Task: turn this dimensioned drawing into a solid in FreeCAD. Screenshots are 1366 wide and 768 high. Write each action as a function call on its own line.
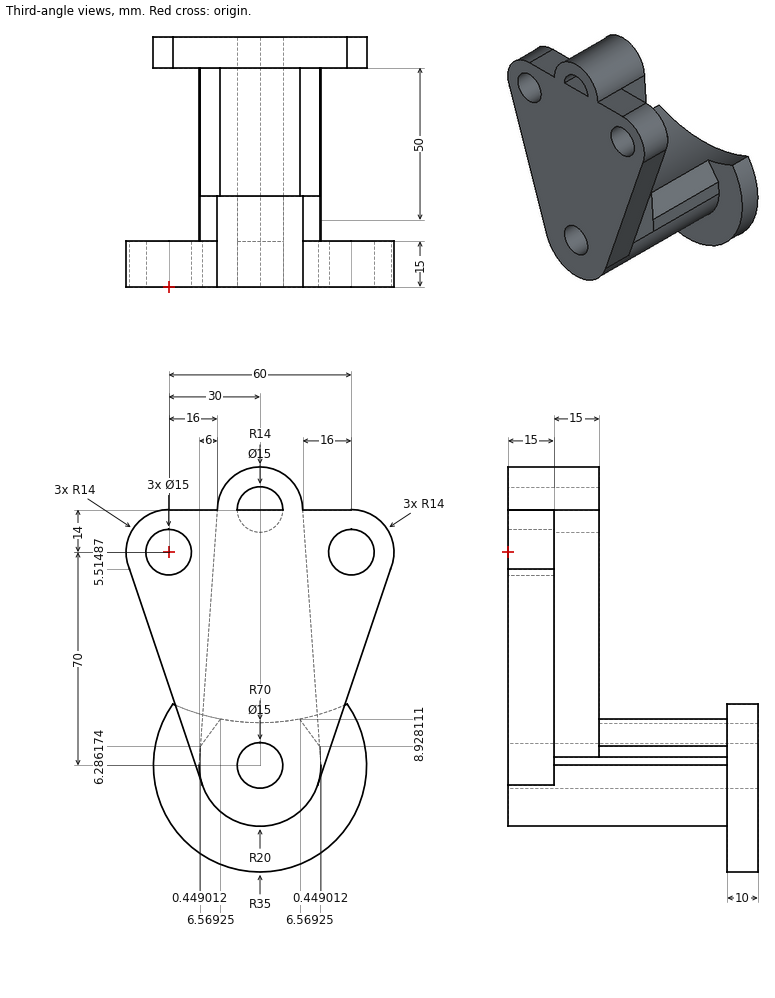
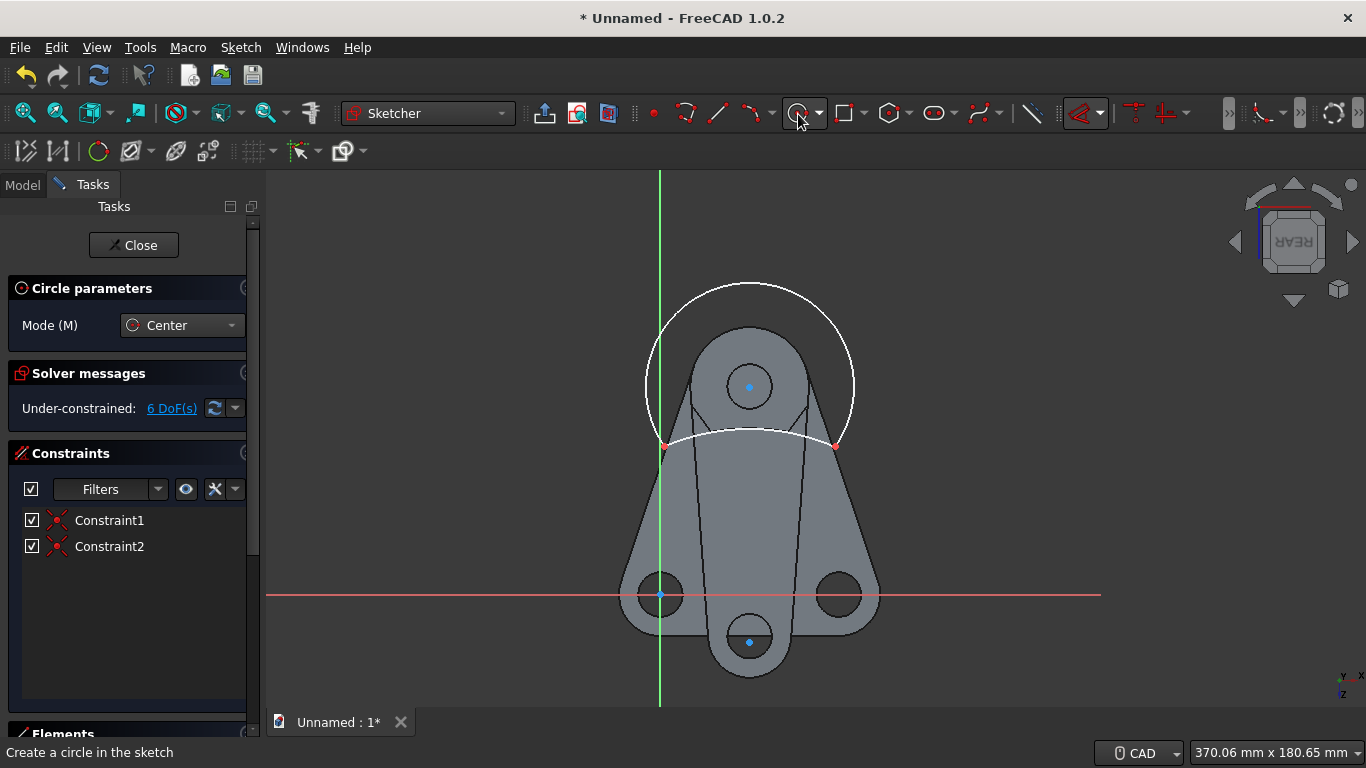
click(750, 387)
move(765, 371)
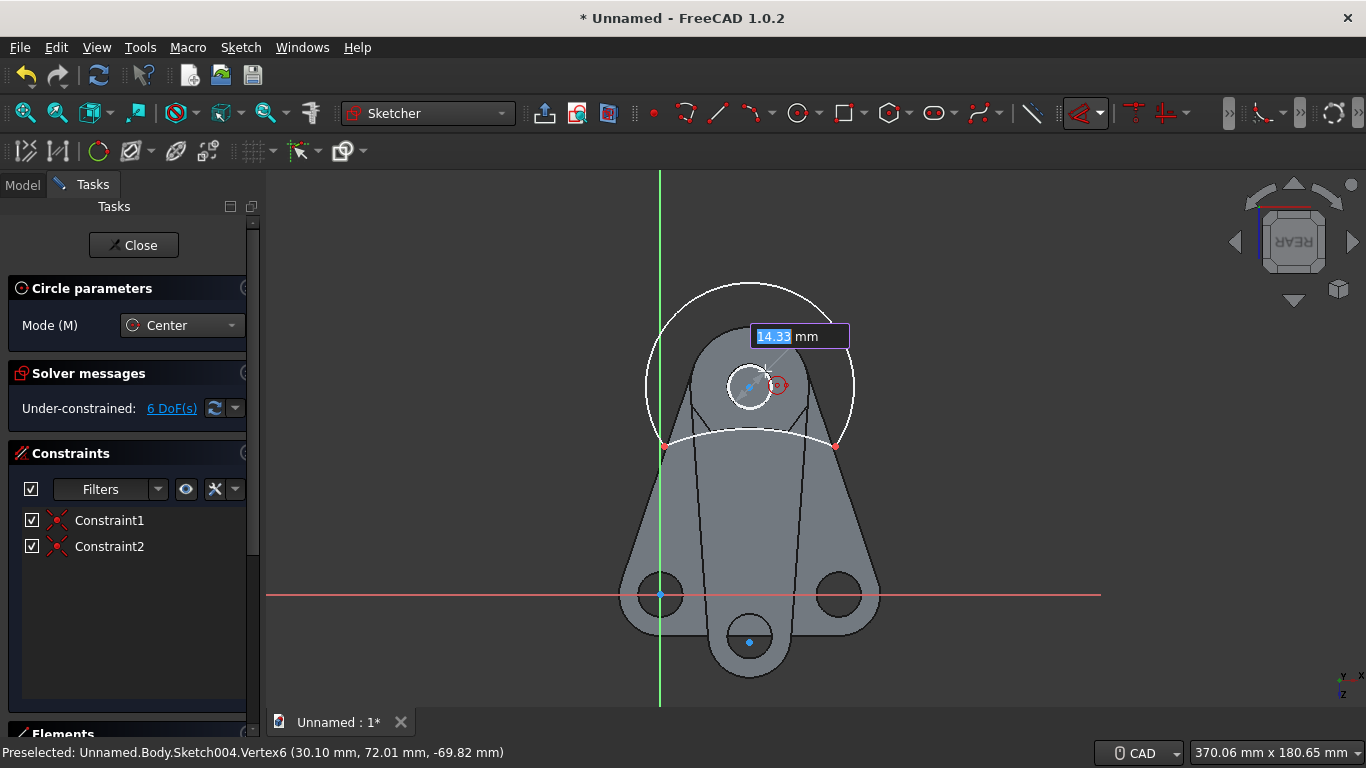
text(15)
key(Return)
key(Escape)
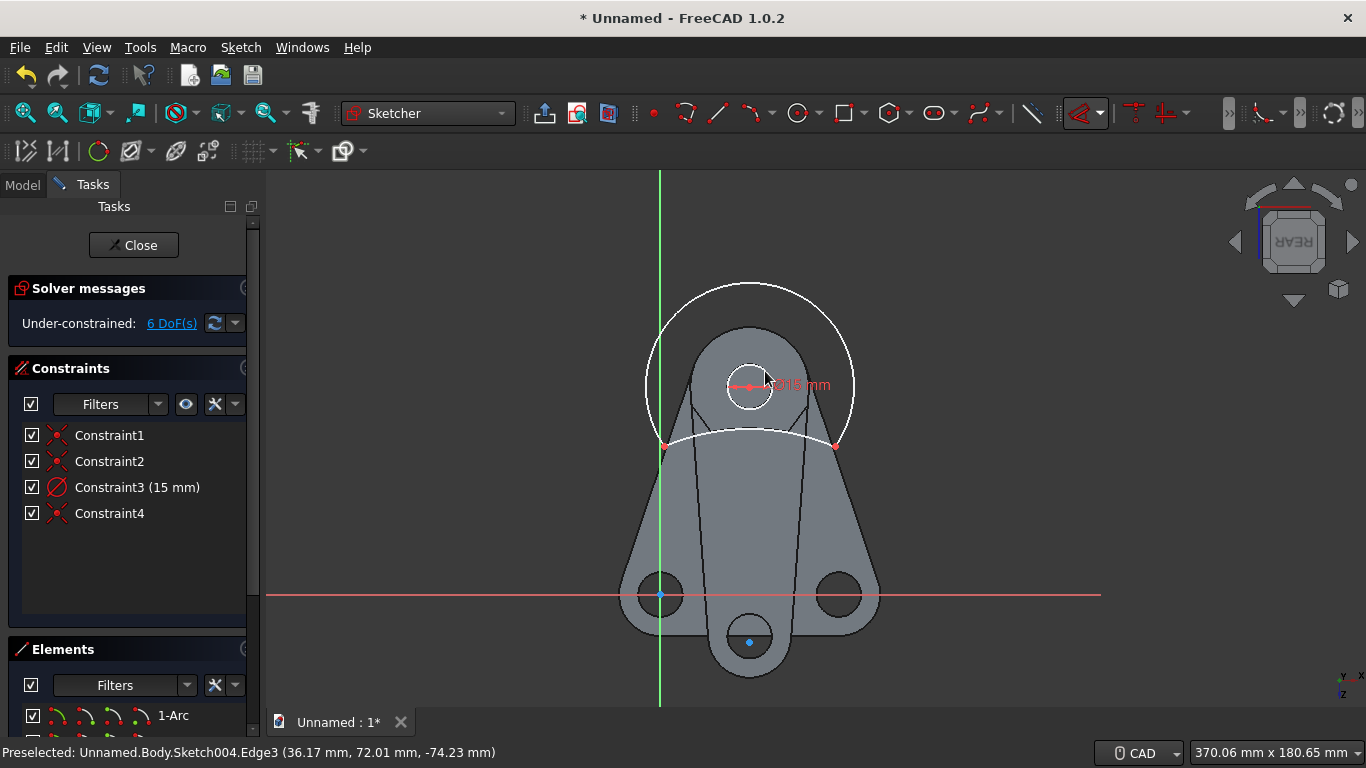
click(785, 432)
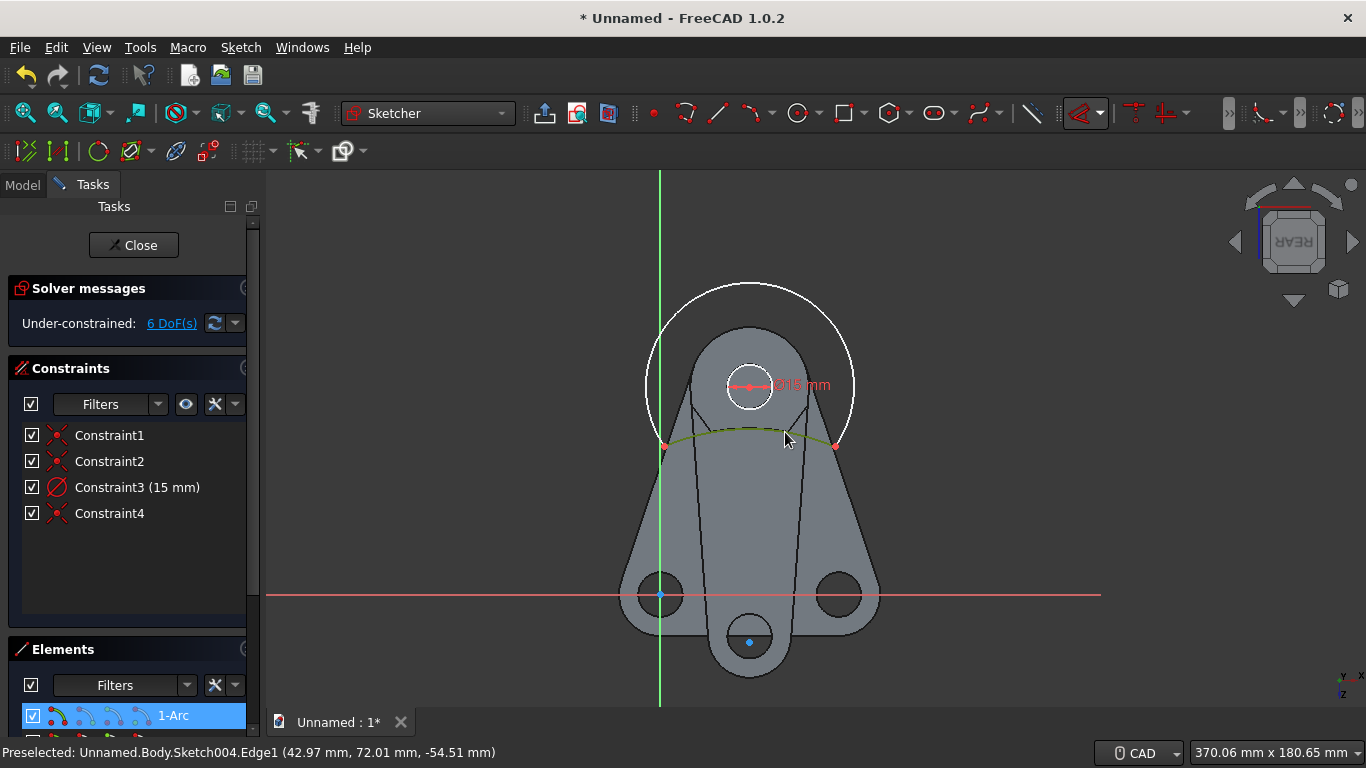
key(k)
key(r)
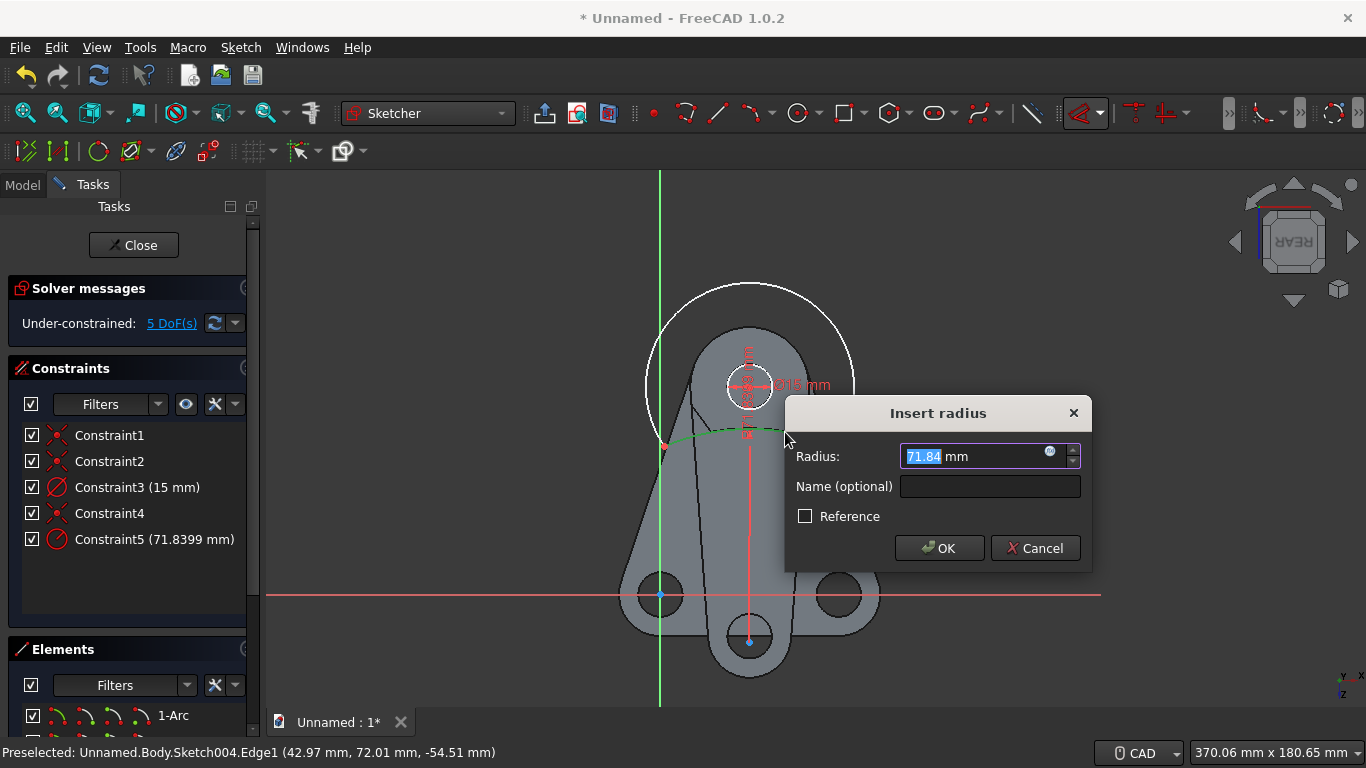
text(70)
key(Return)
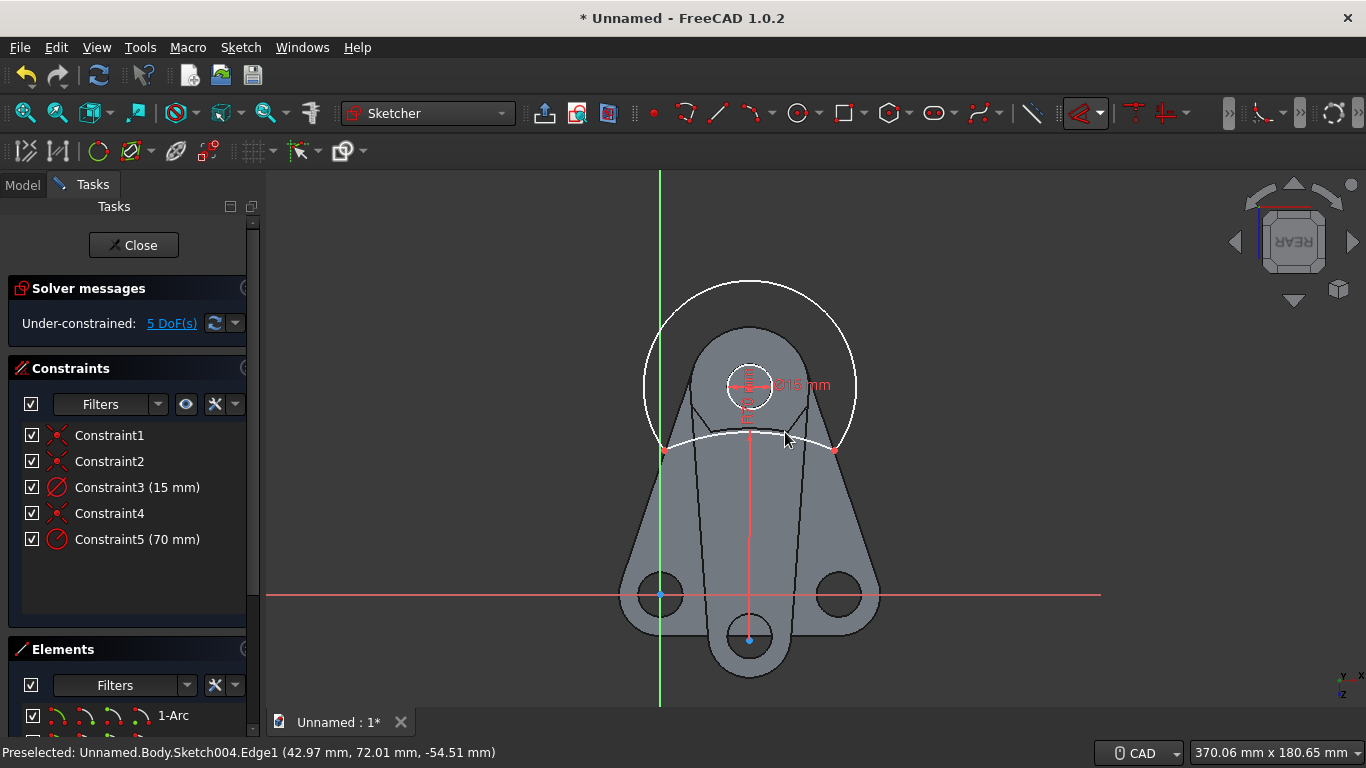
click(832, 320)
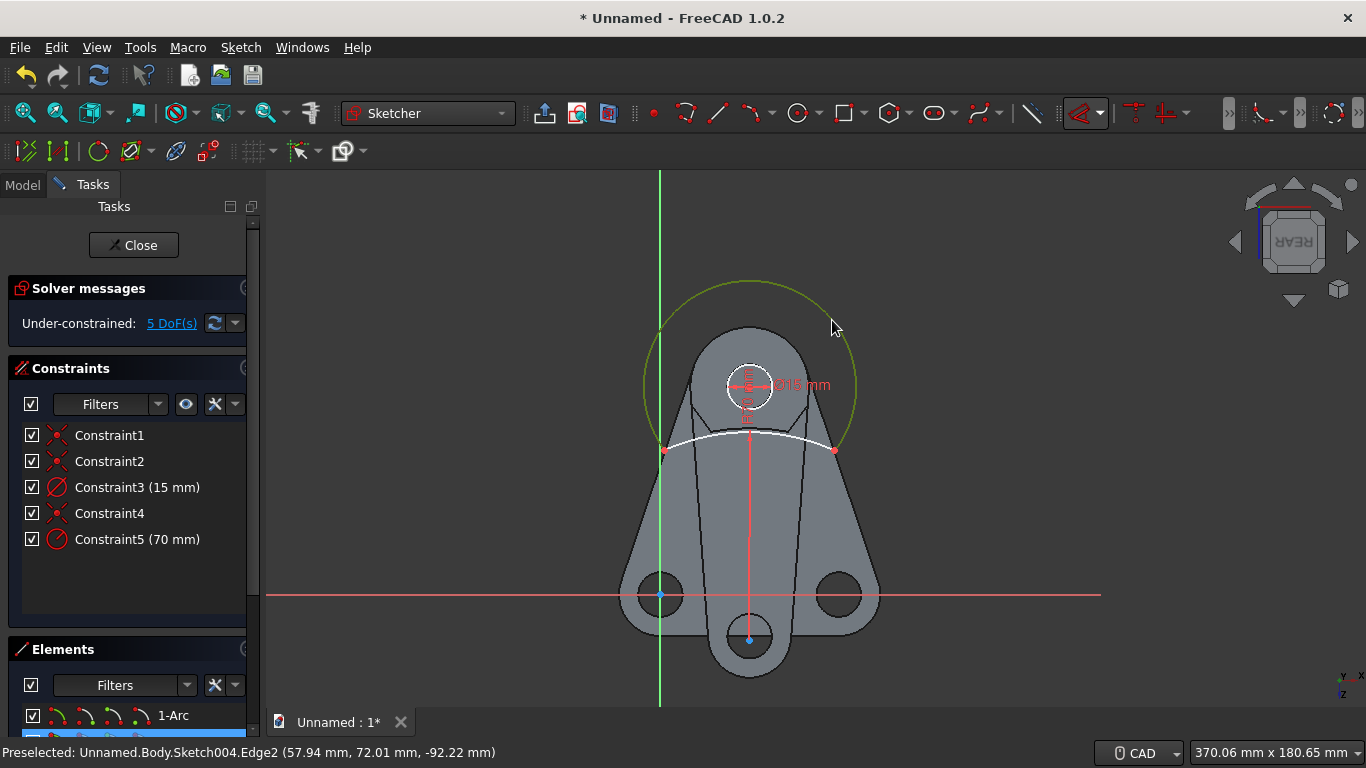
key(k)
key(r)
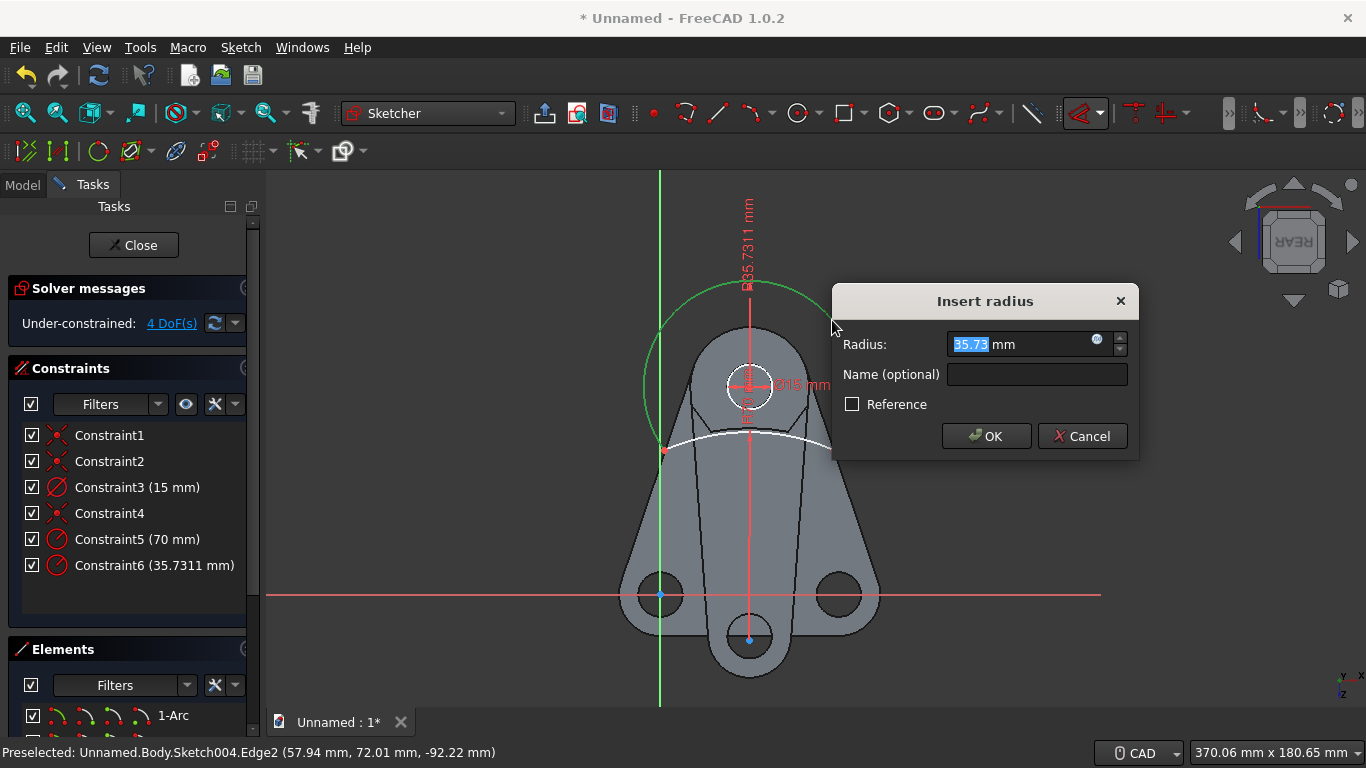
text(35)
key(Return)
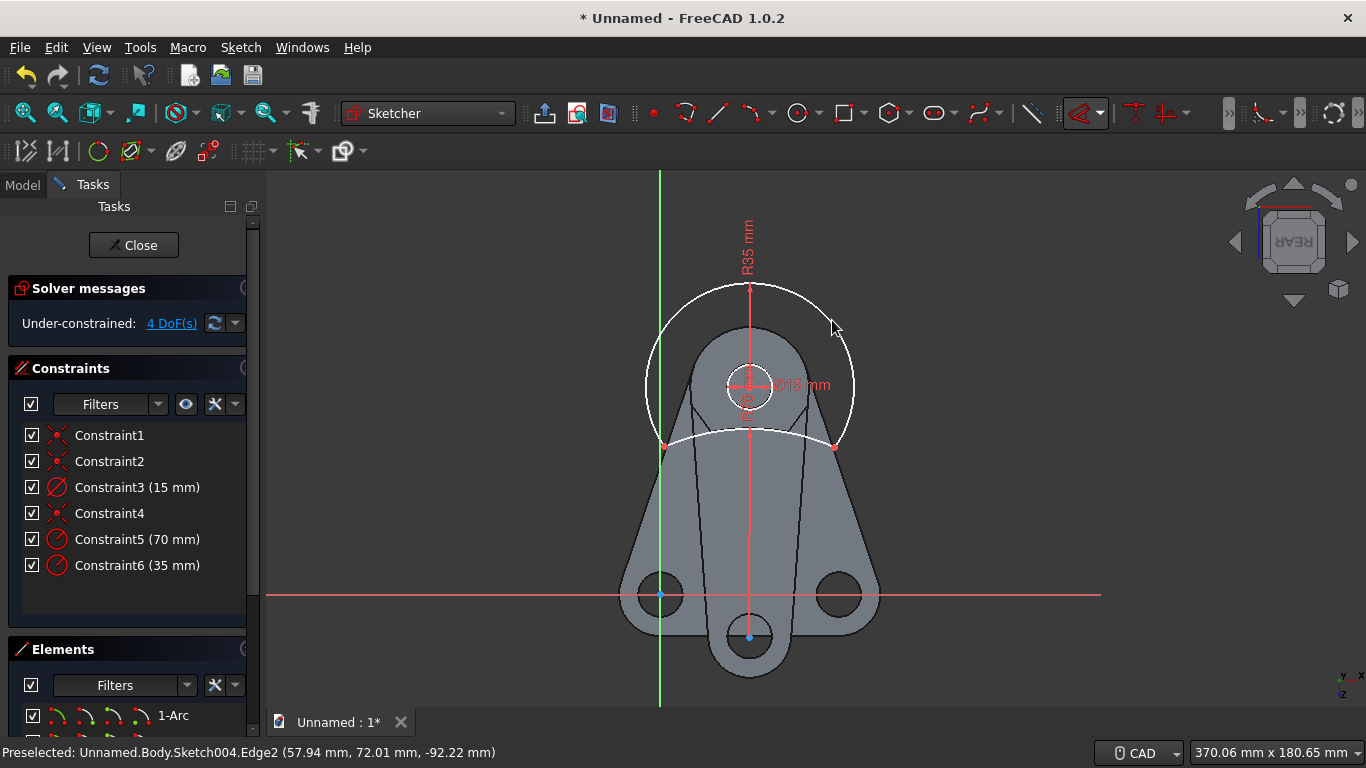
click(750, 387)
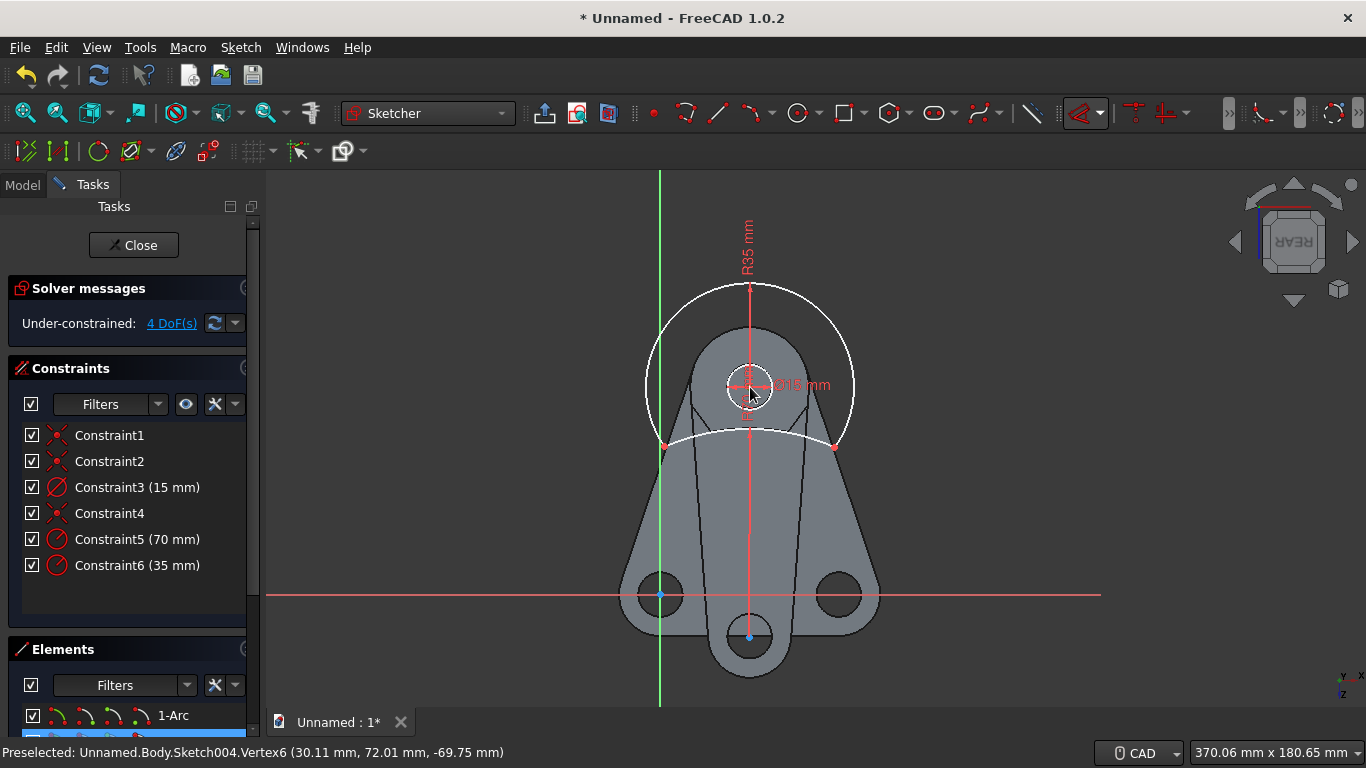
click(1102, 114)